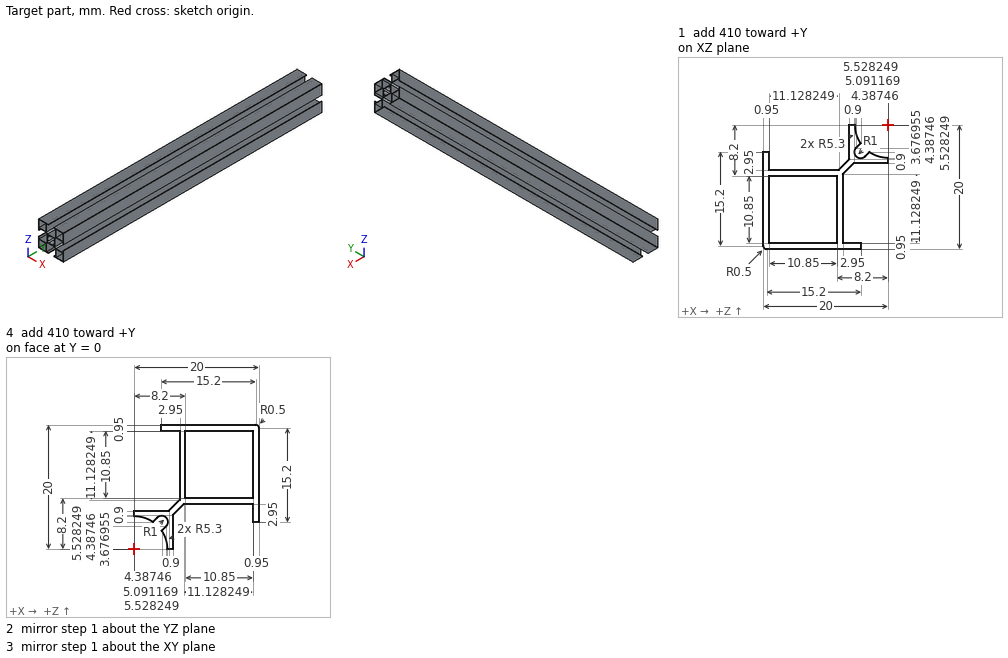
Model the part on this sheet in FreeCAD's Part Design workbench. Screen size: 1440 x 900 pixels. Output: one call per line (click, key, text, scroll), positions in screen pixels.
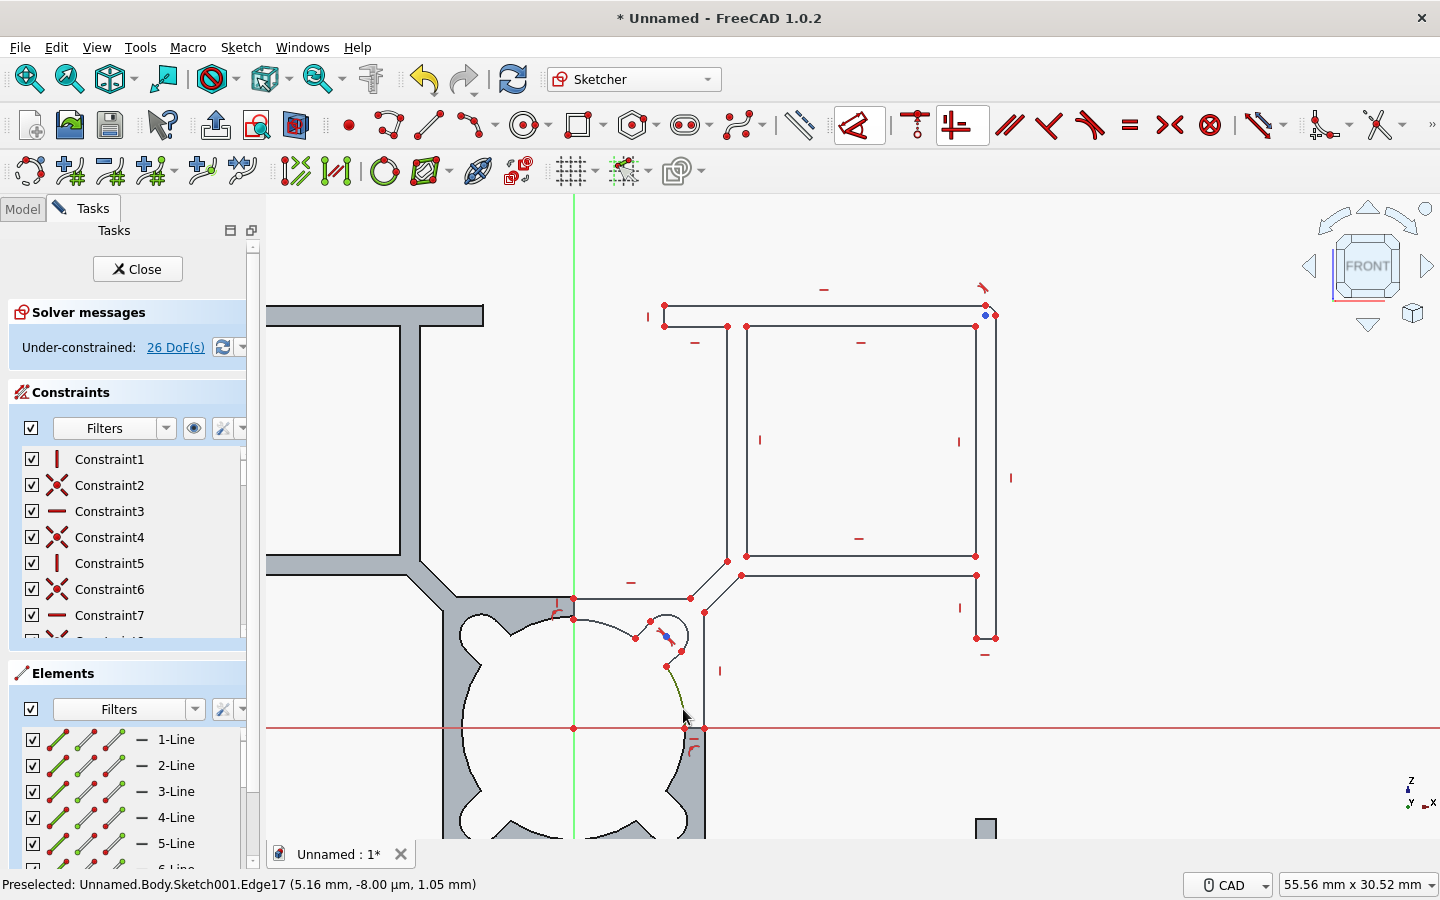
click(618, 629)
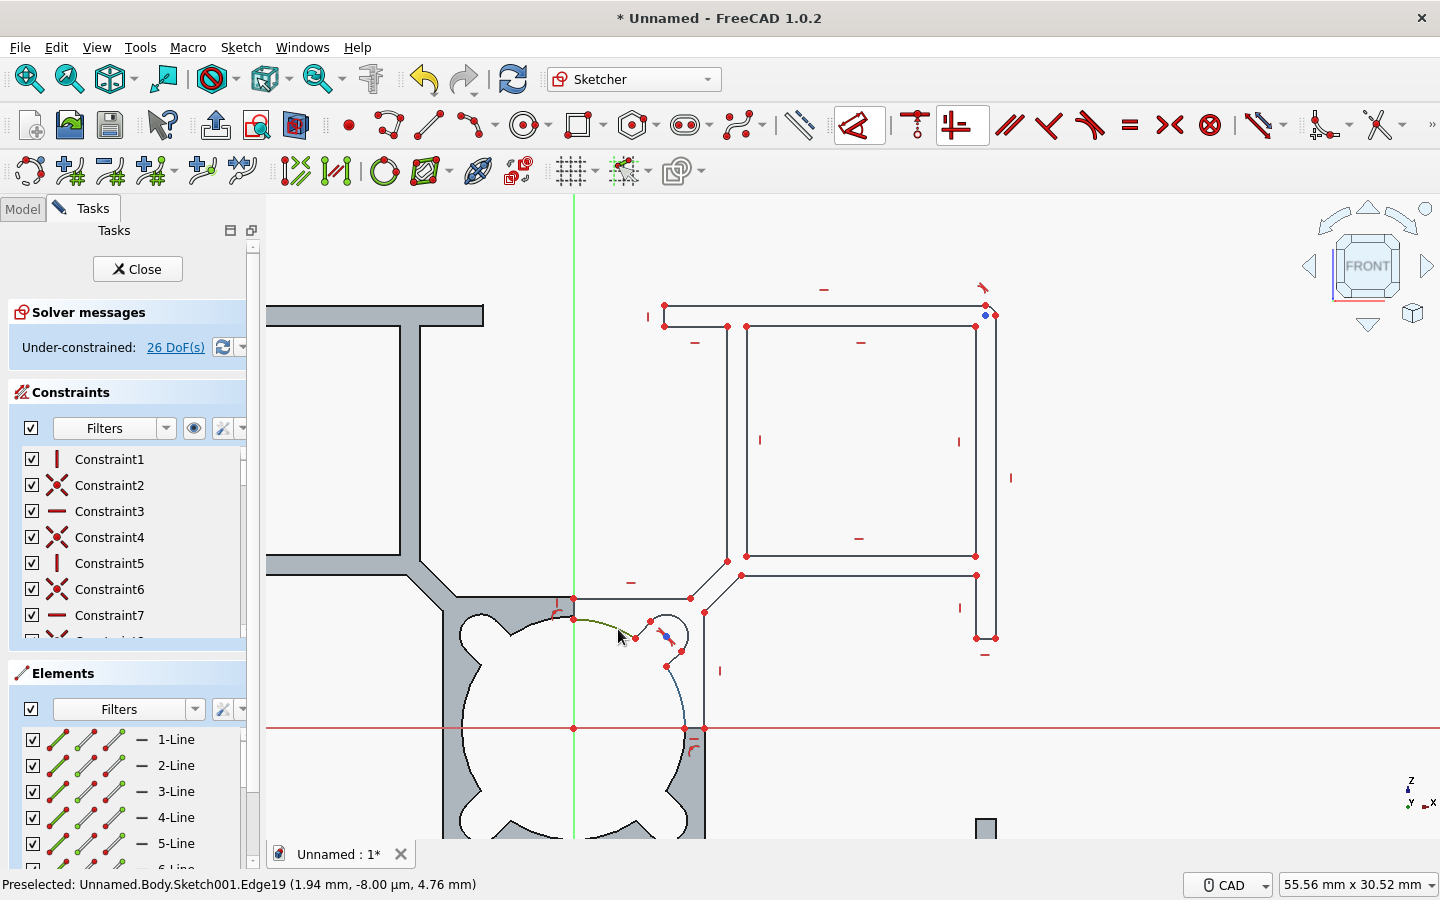
key(e)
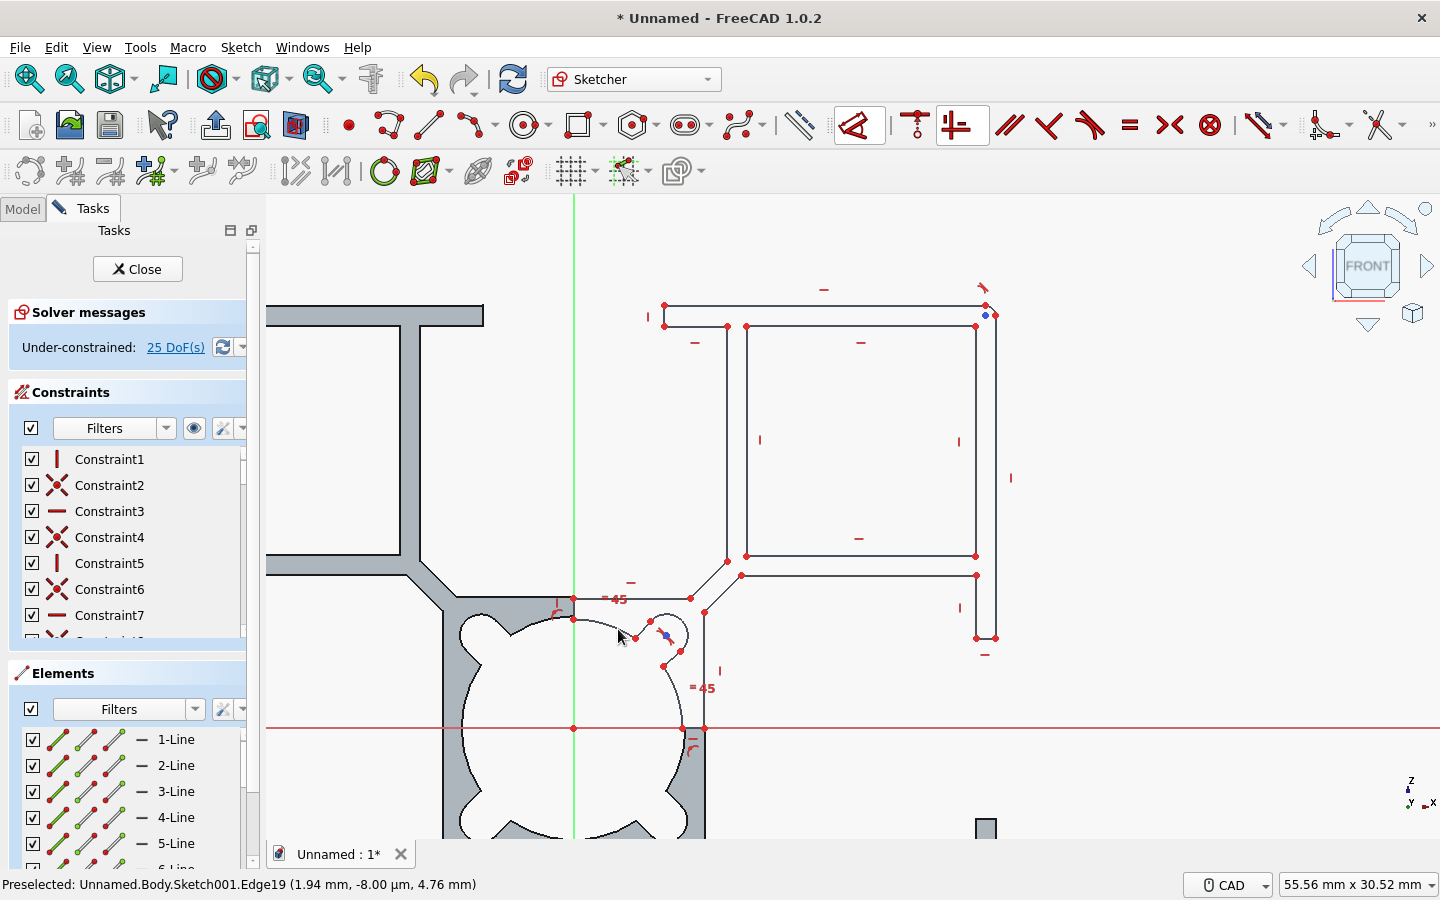
click(680, 709)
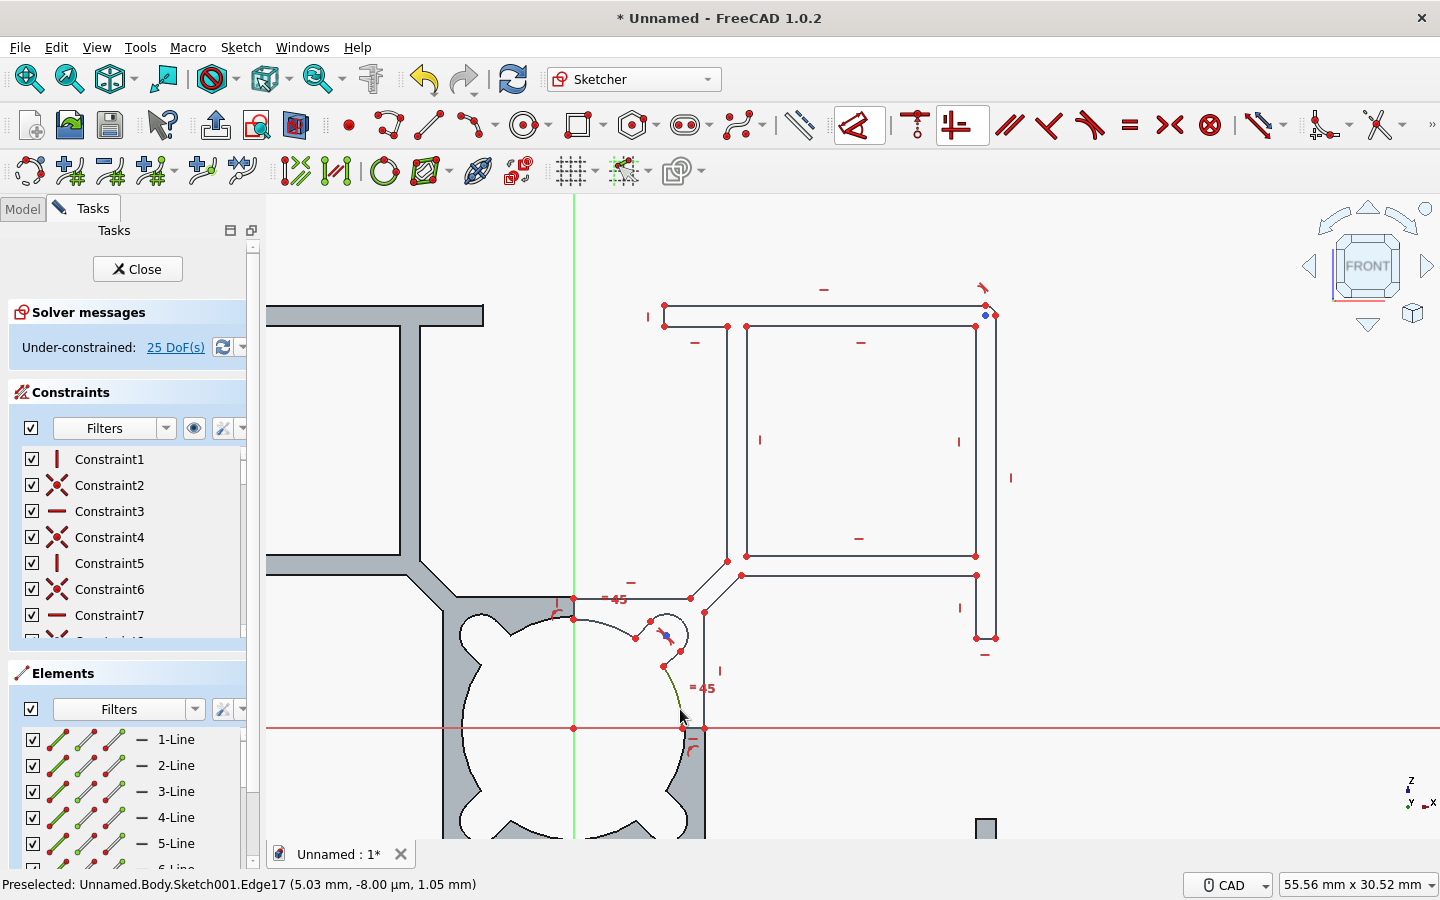
click(880, 126)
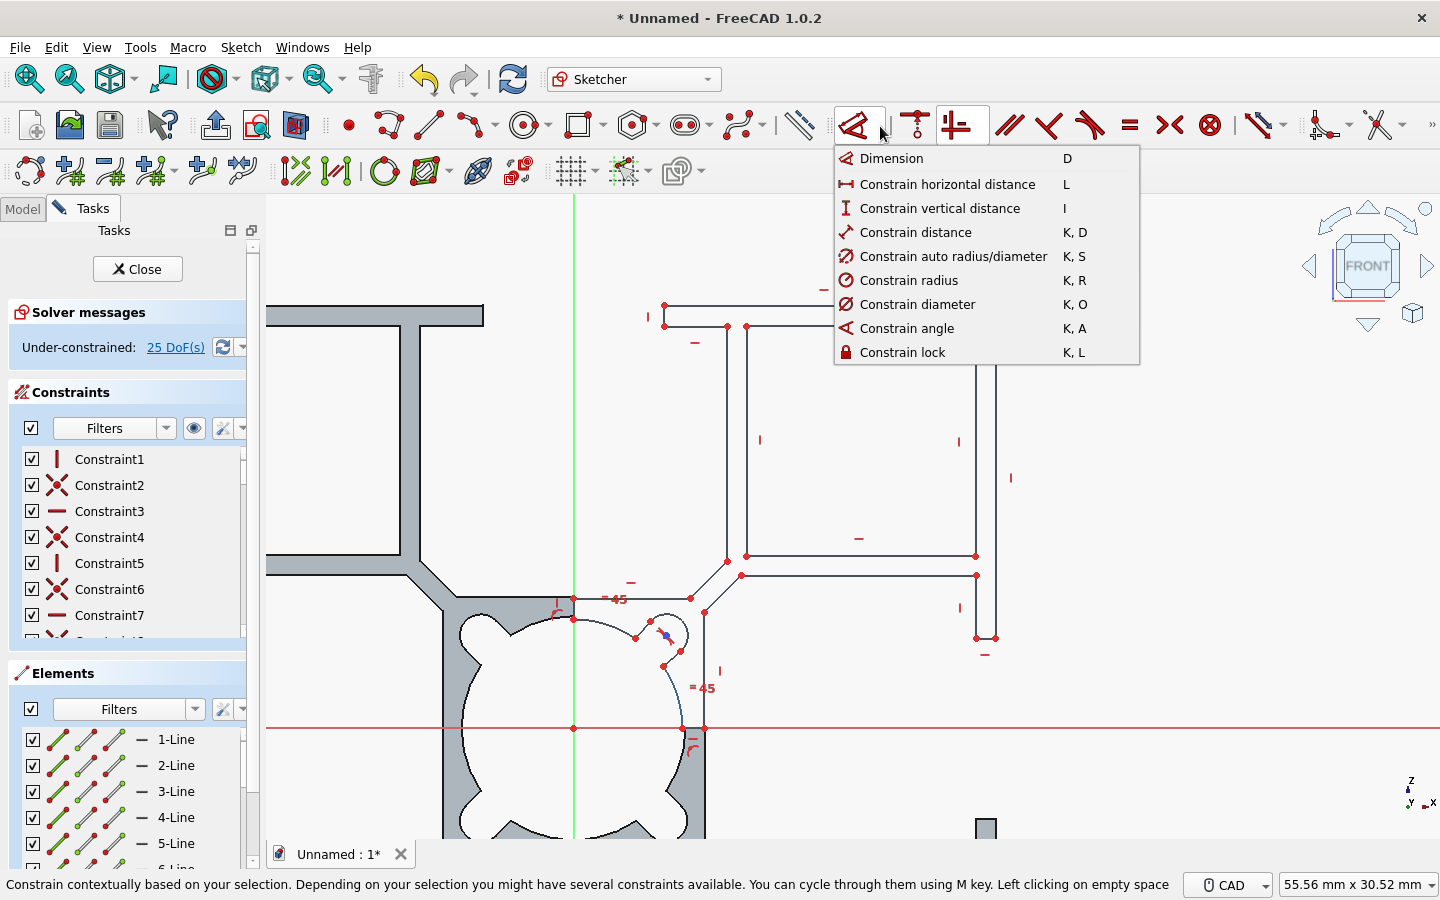
click(987, 280)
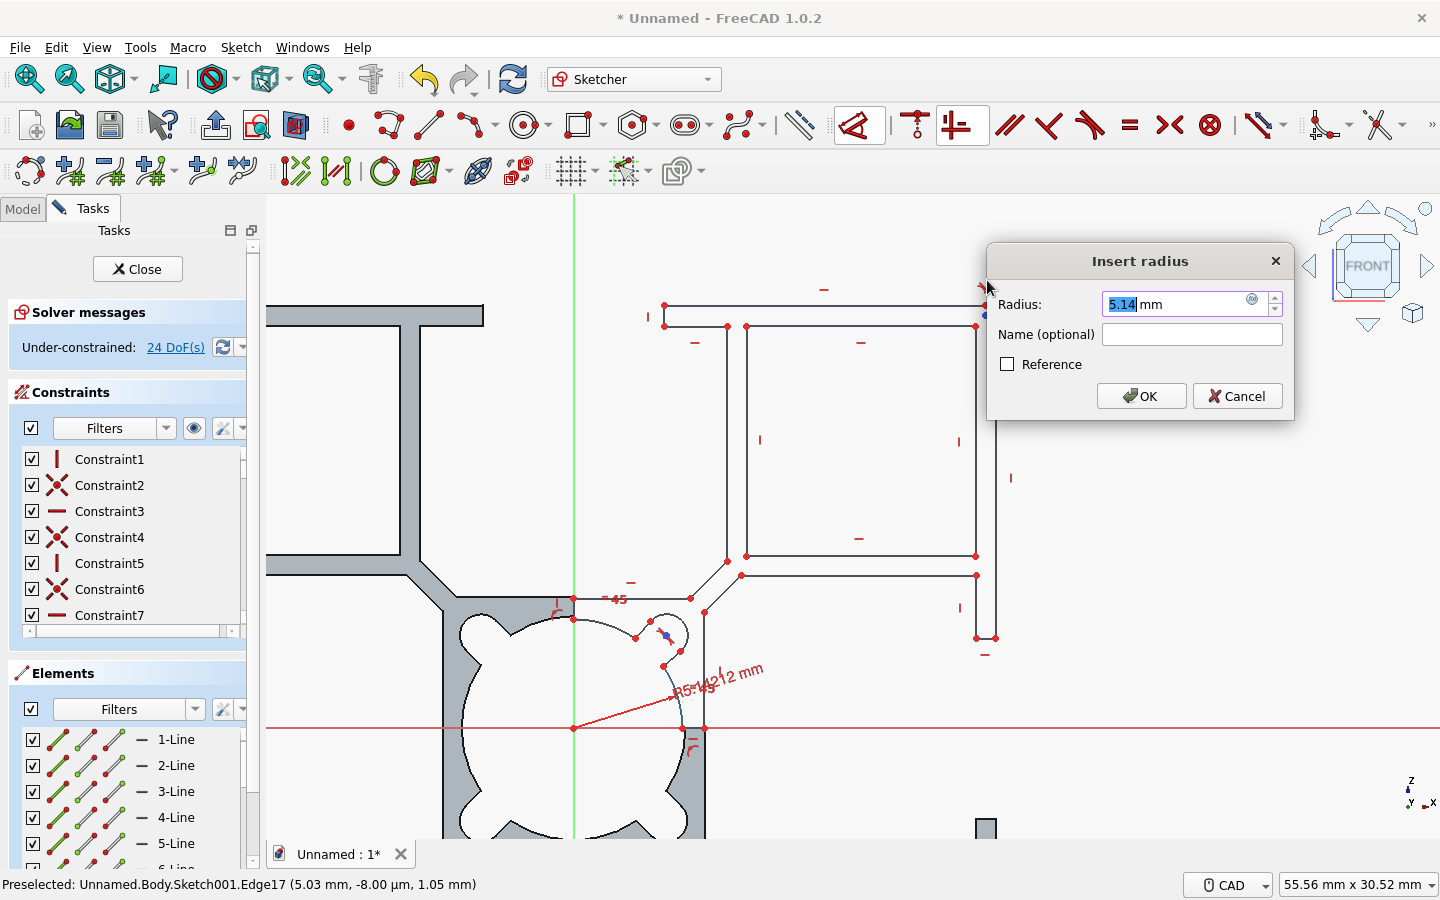
text(5.3)
key(Return)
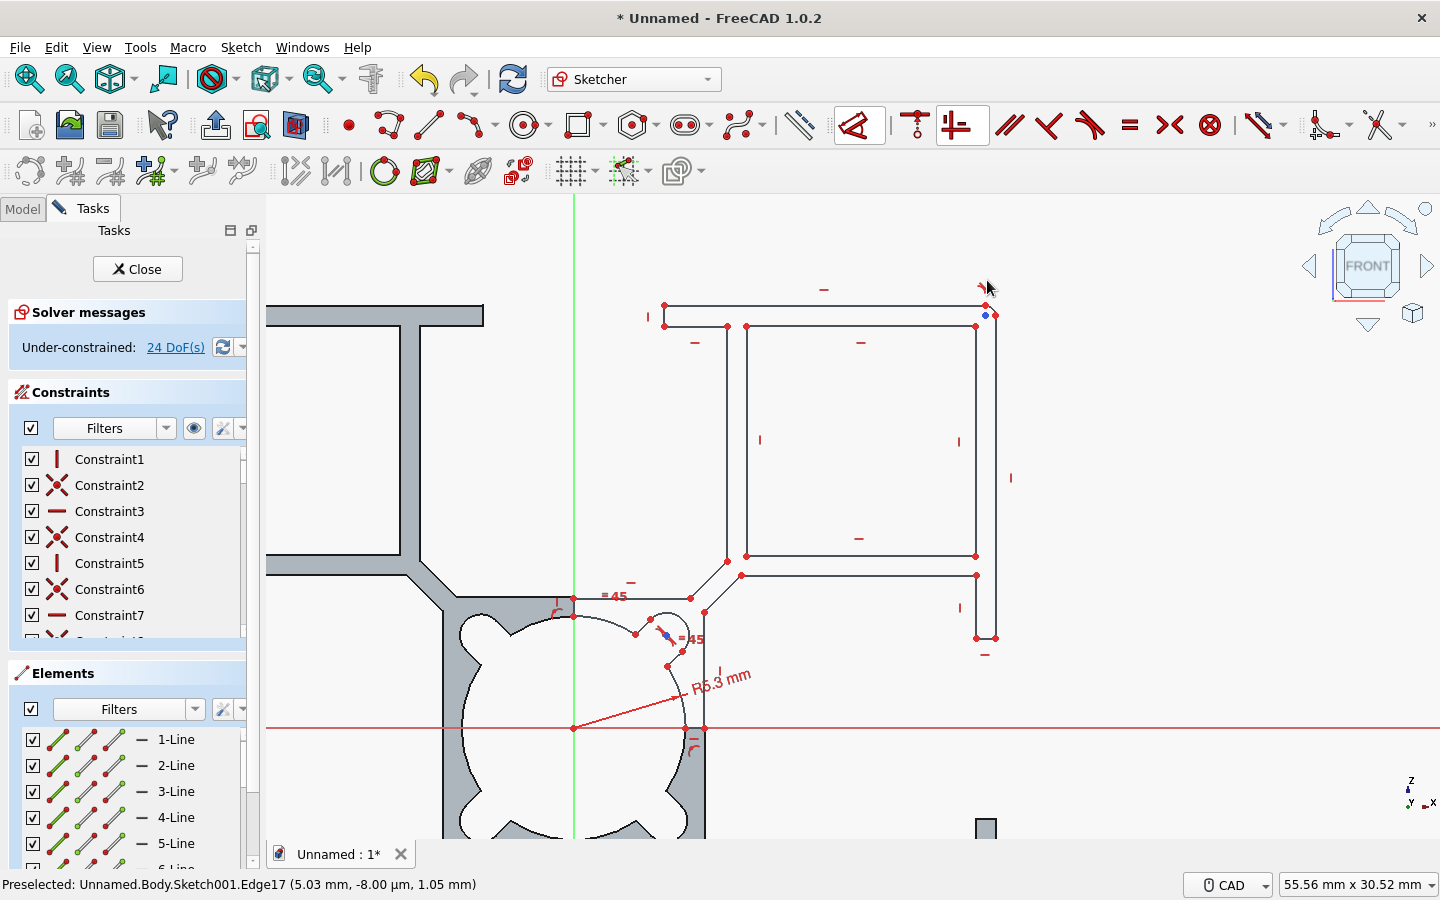
scroll(689, 632, up, 4)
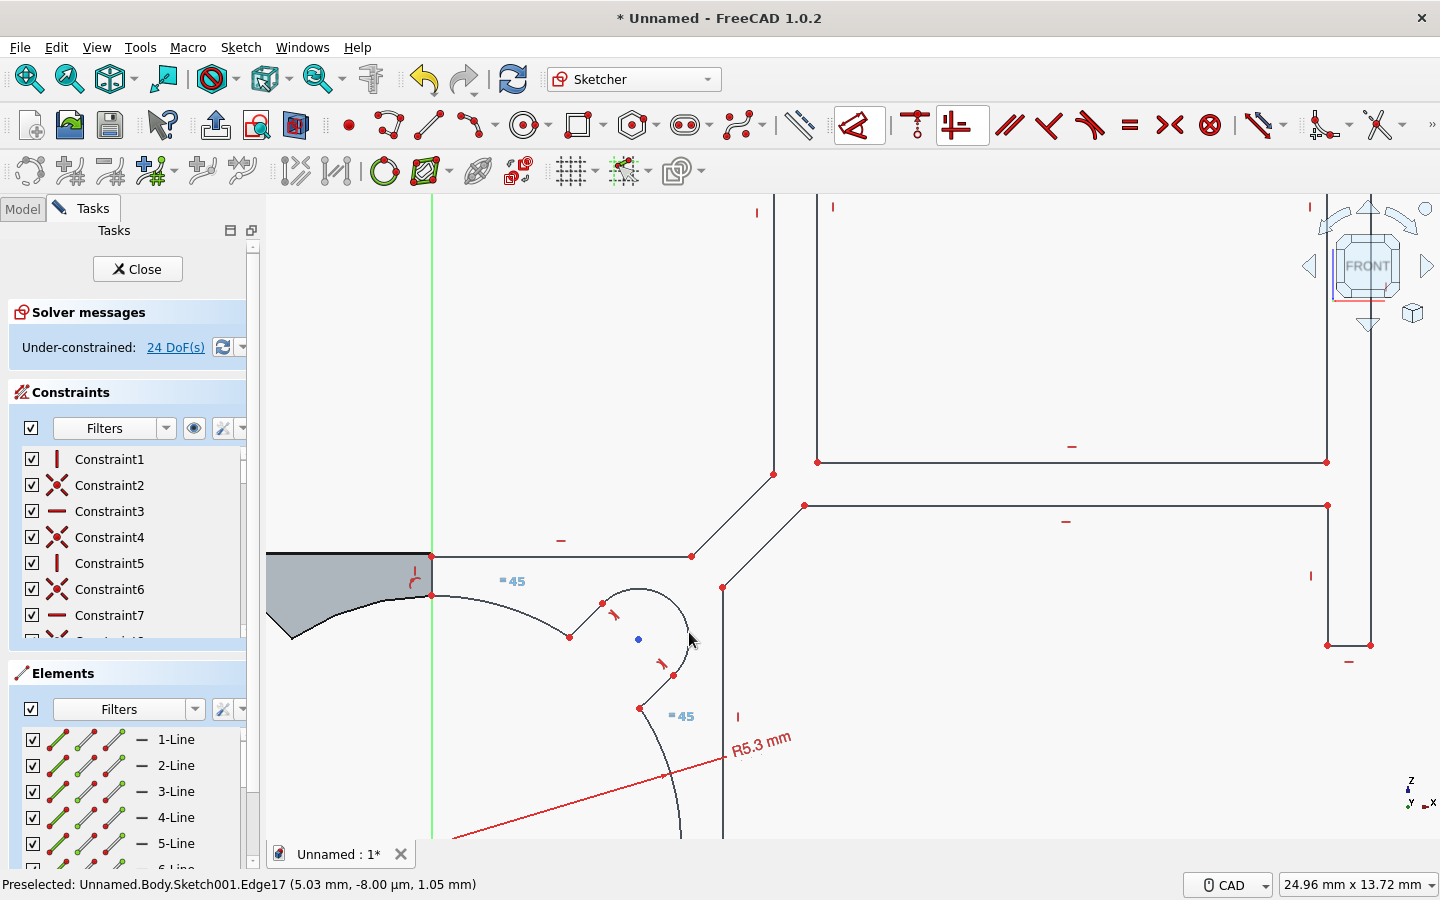
click(688, 632)